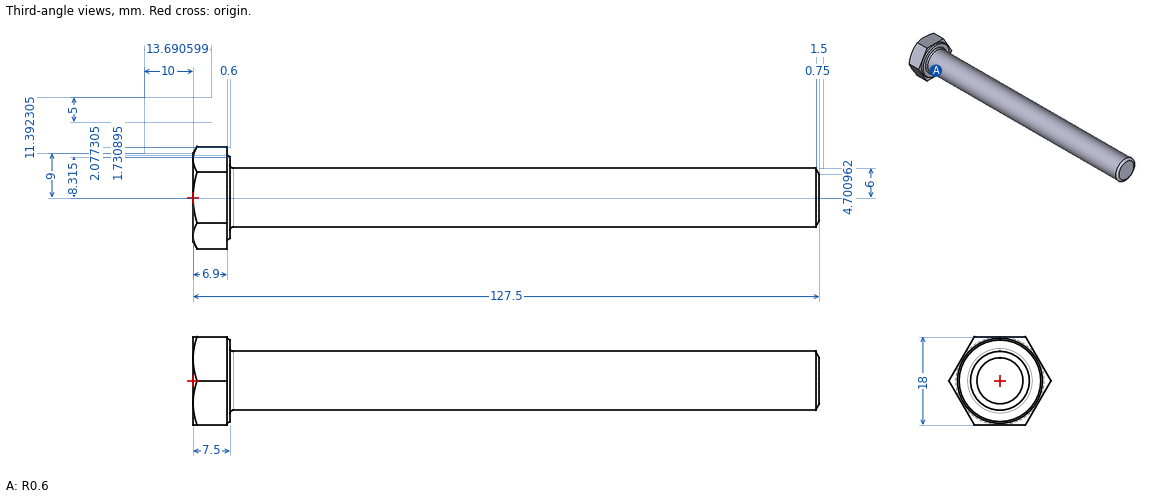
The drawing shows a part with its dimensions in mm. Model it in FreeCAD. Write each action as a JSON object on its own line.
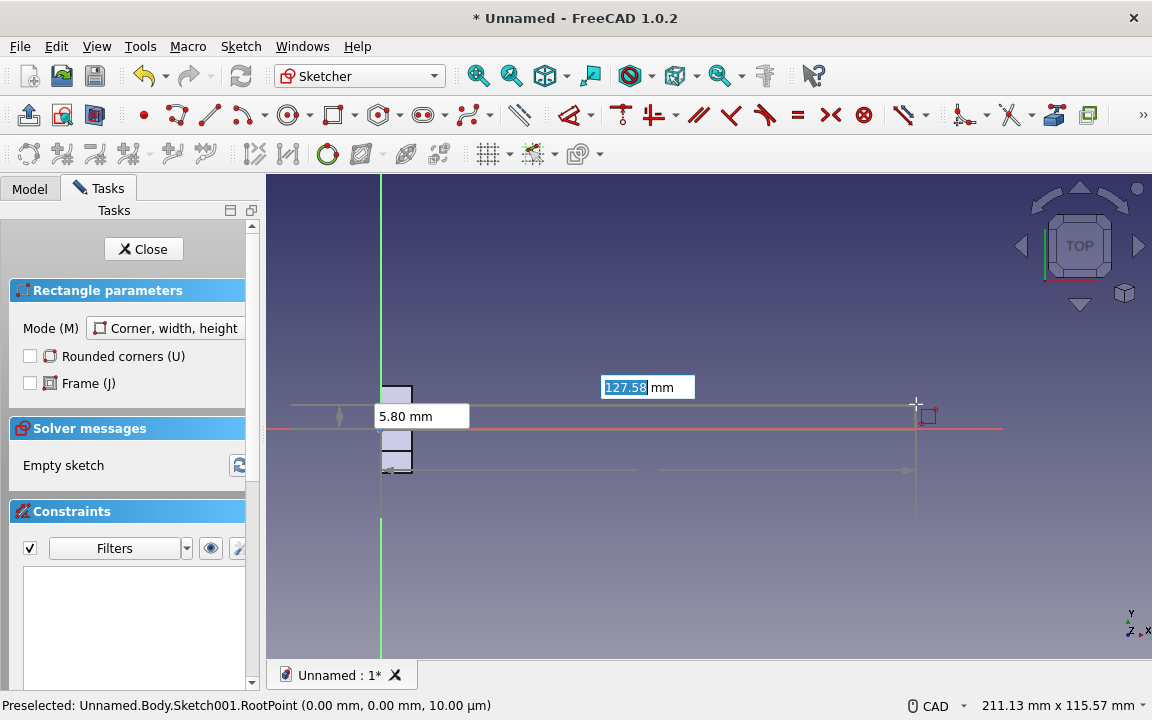
{"action": "type", "text": "127.5"}
{"action": "key", "text": "Tab"}
{"action": "type", "text": "6"}
{"action": "key", "text": "Return"}
{"action": "key", "text": "Escape"}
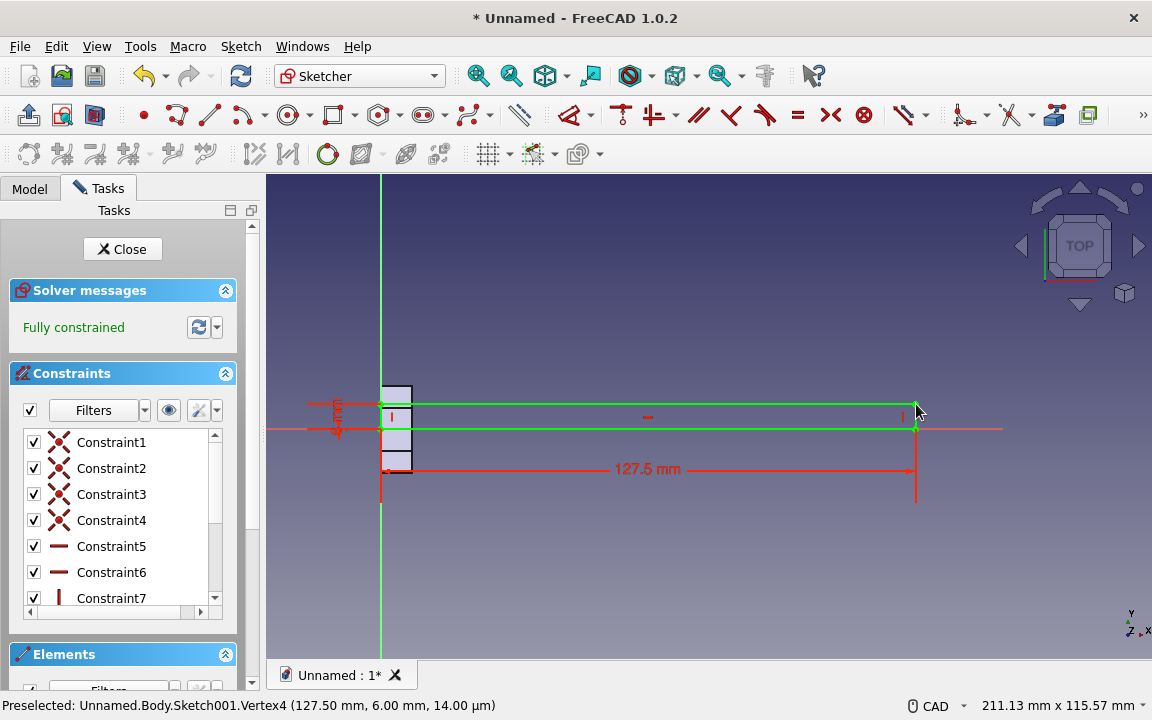
{"action": "left_click", "coordinate": [123, 249]}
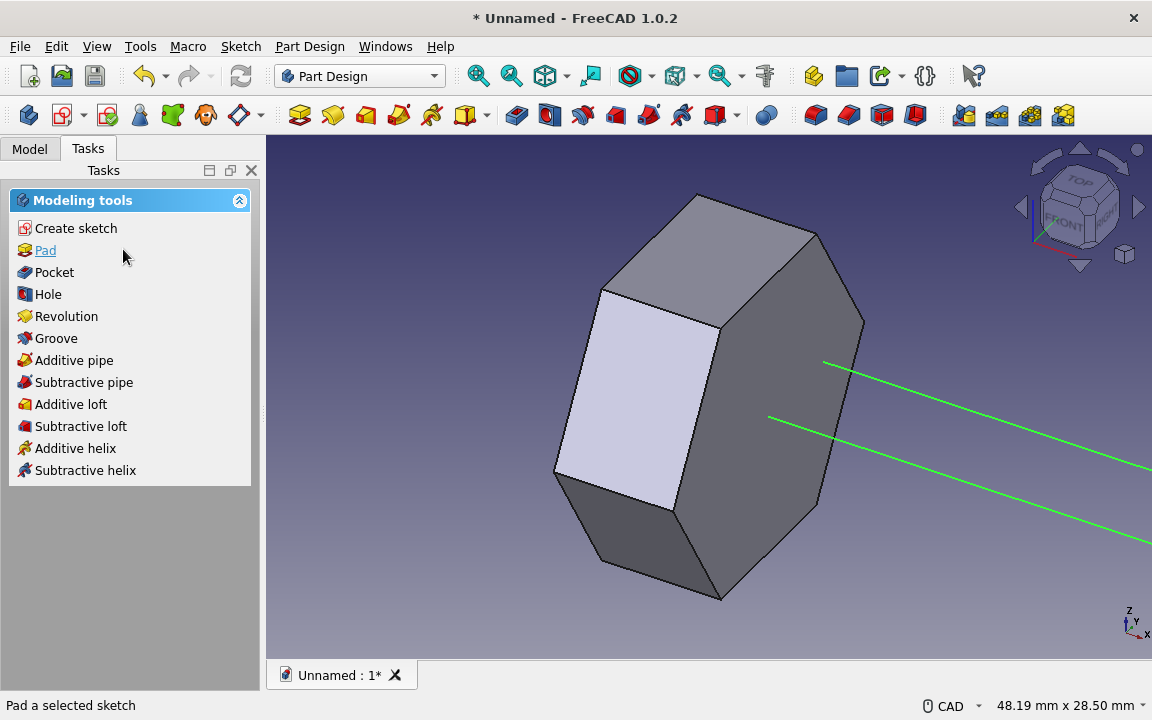
{"action": "left_click", "coordinate": [333, 116]}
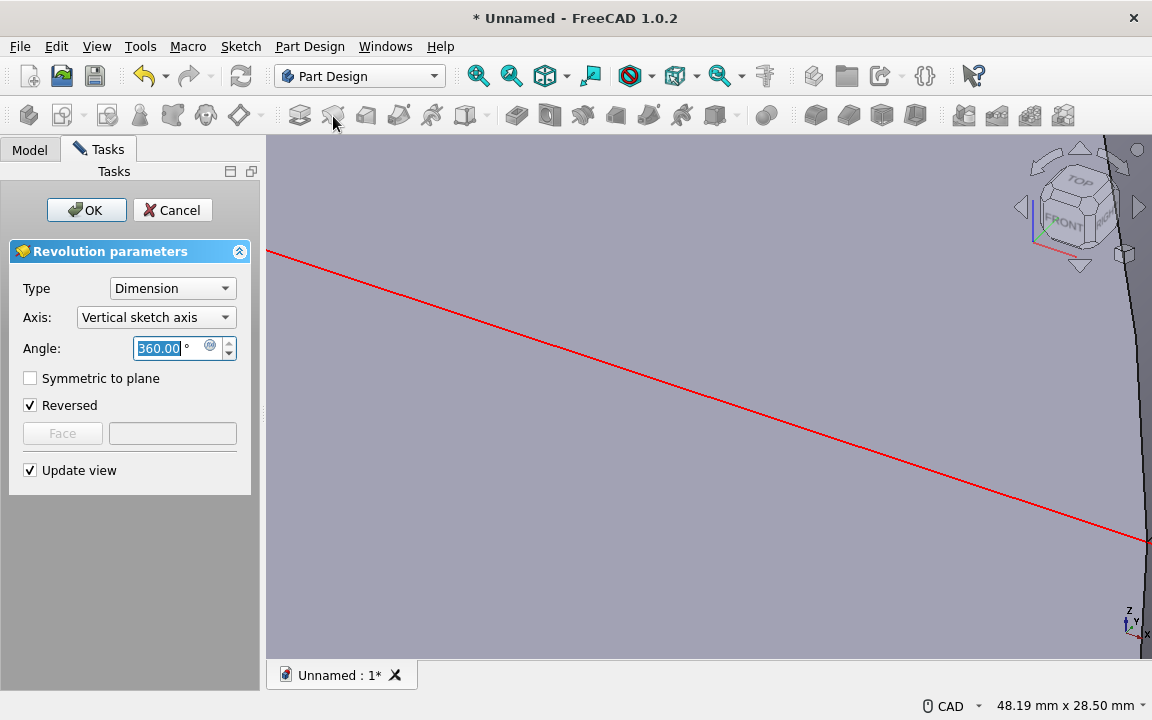
{"action": "left_click", "coordinate": [157, 318]}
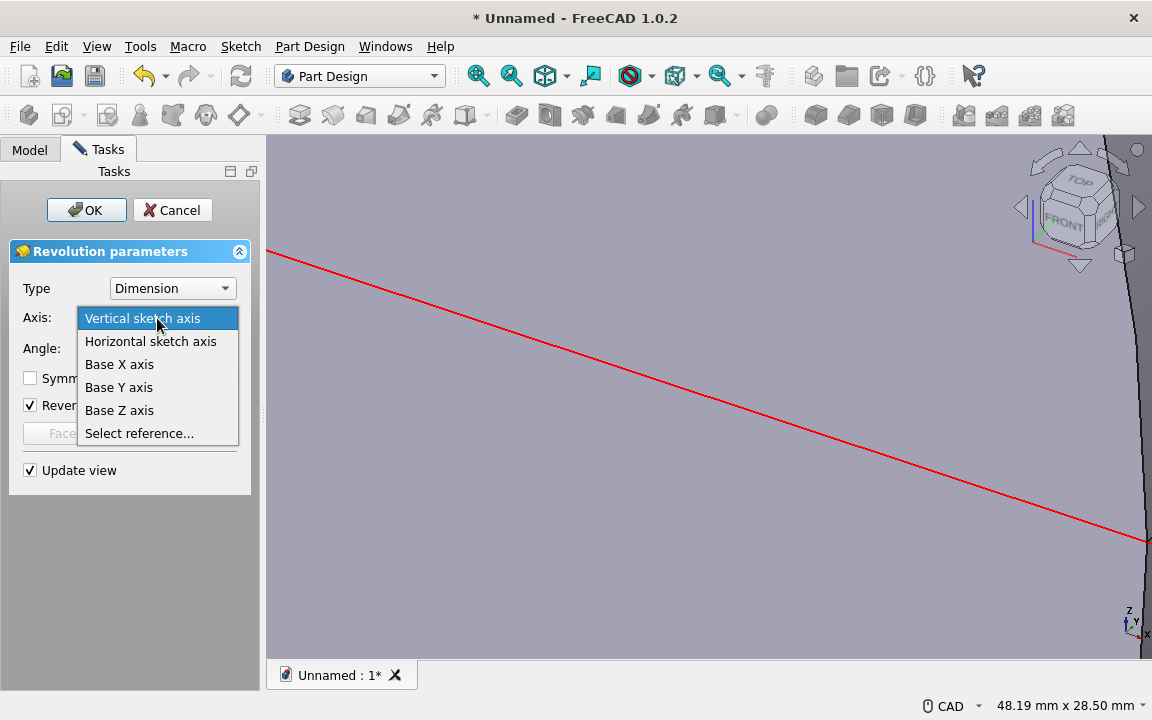
{"action": "left_click", "coordinate": [156, 342]}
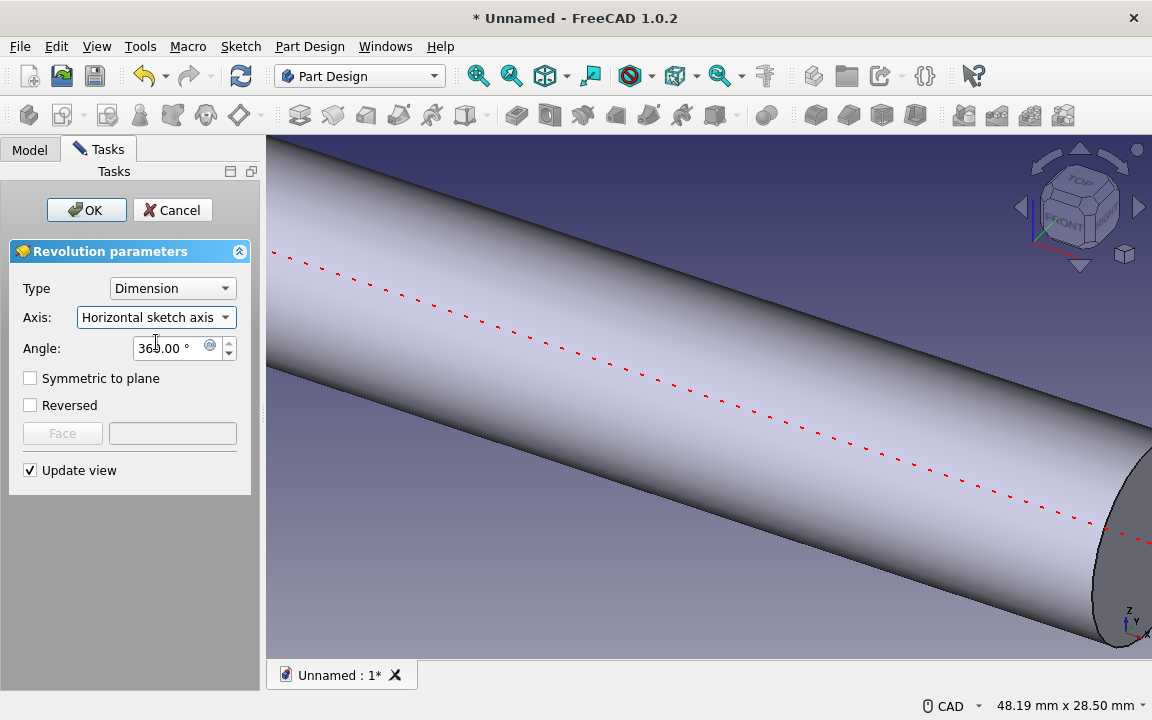
{"action": "left_click", "coordinate": [87, 210]}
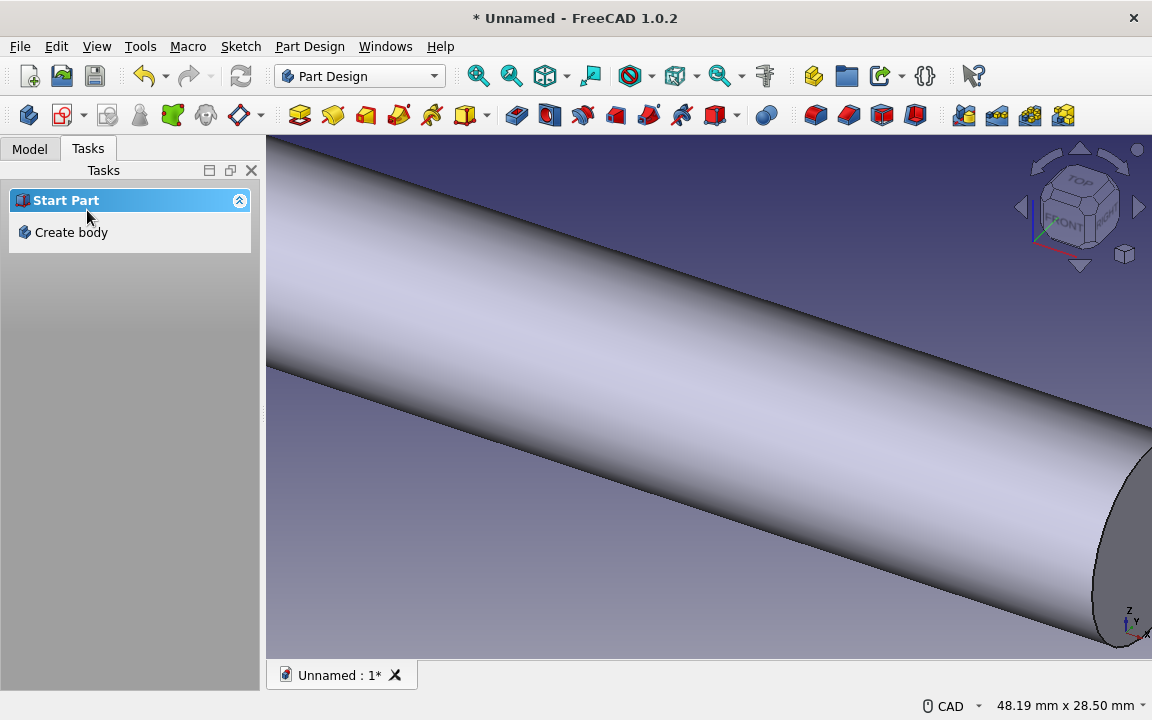
{"action": "left_click", "coordinate": [479, 76]}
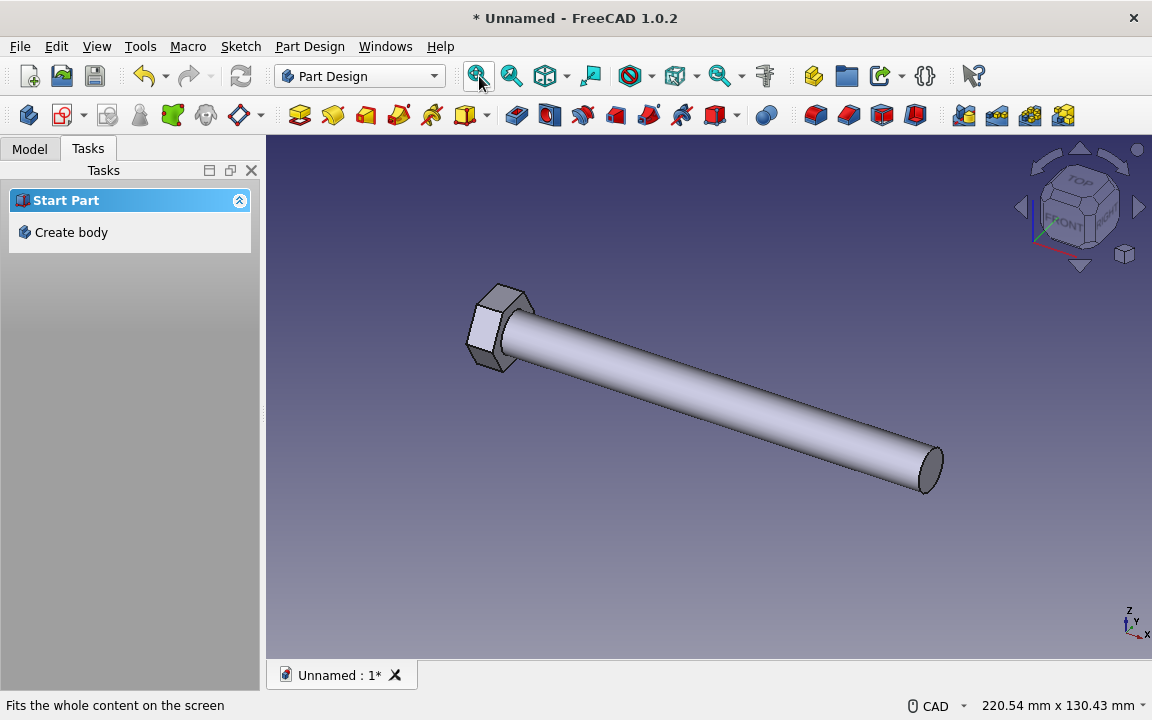
{"action": "left_click", "coordinate": [62, 116]}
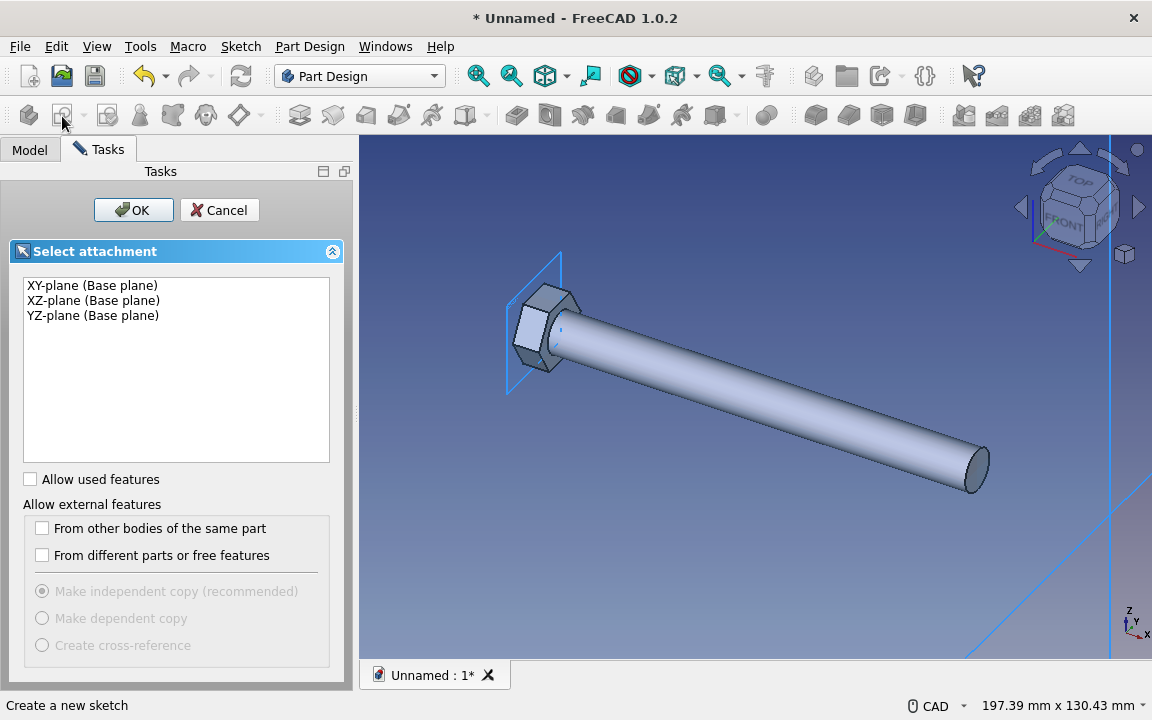
{"action": "left_click", "coordinate": [84, 286]}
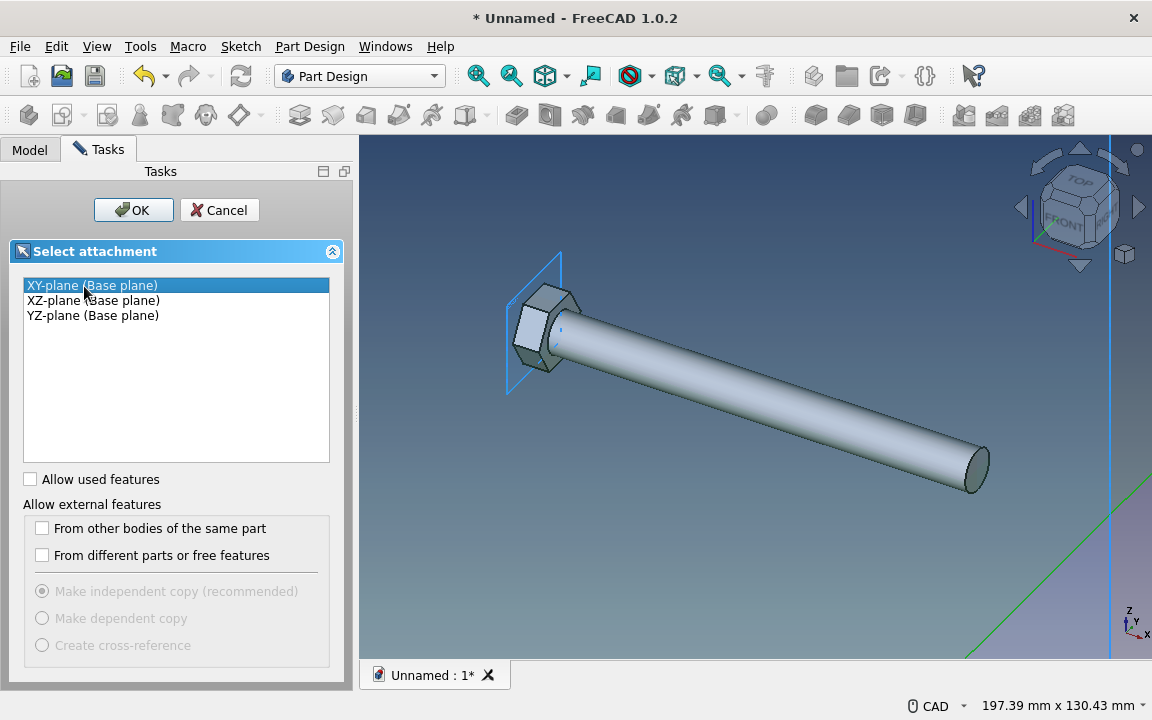
{"action": "left_click", "coordinate": [134, 210]}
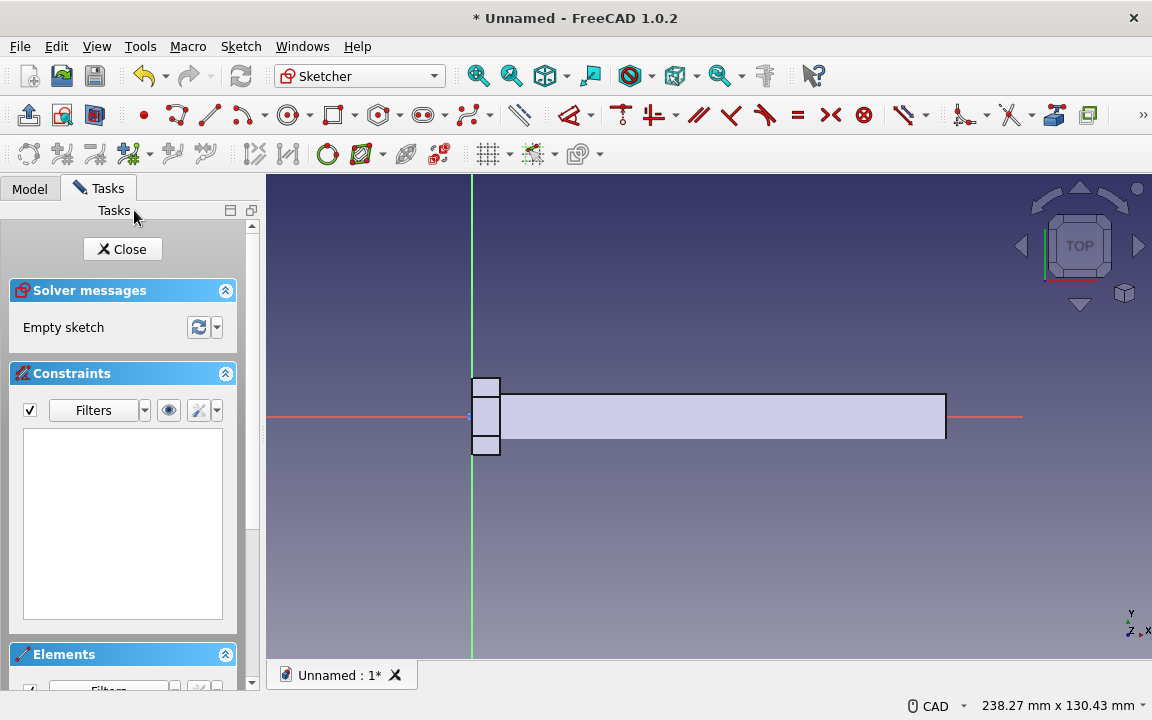
{"action": "left_click", "coordinate": [95, 116]}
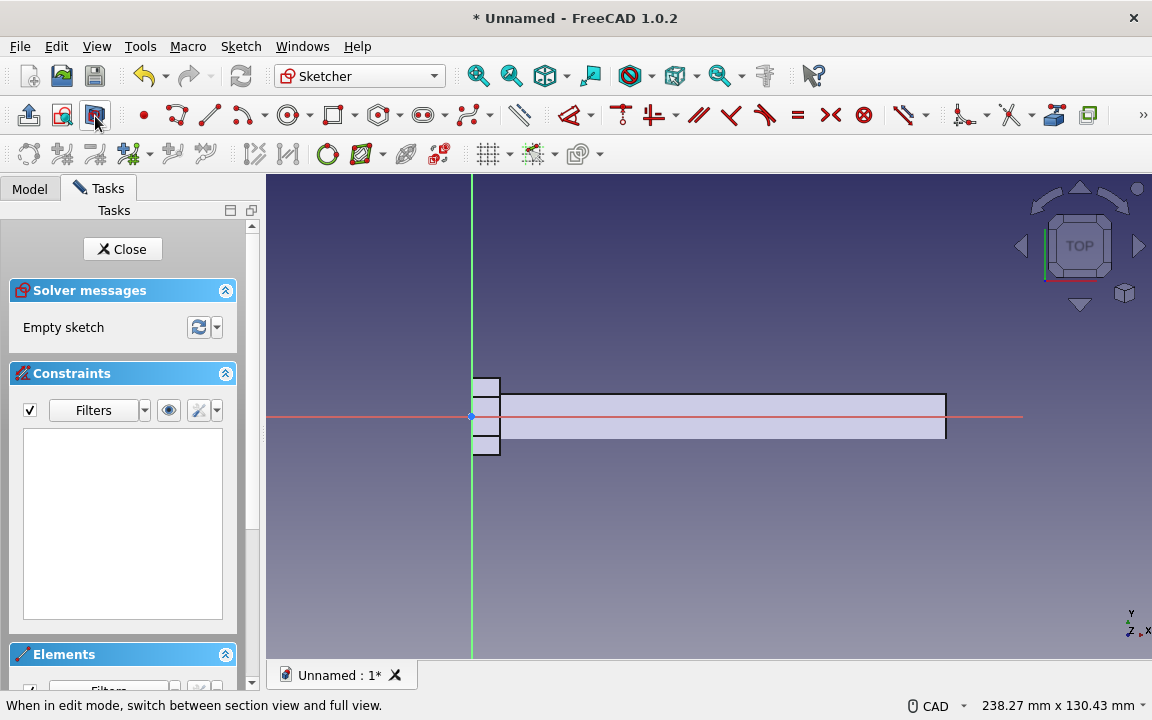
{"action": "scroll", "coordinate": [401, 366], "scroll_direction": "up", "scroll_amount": 7}